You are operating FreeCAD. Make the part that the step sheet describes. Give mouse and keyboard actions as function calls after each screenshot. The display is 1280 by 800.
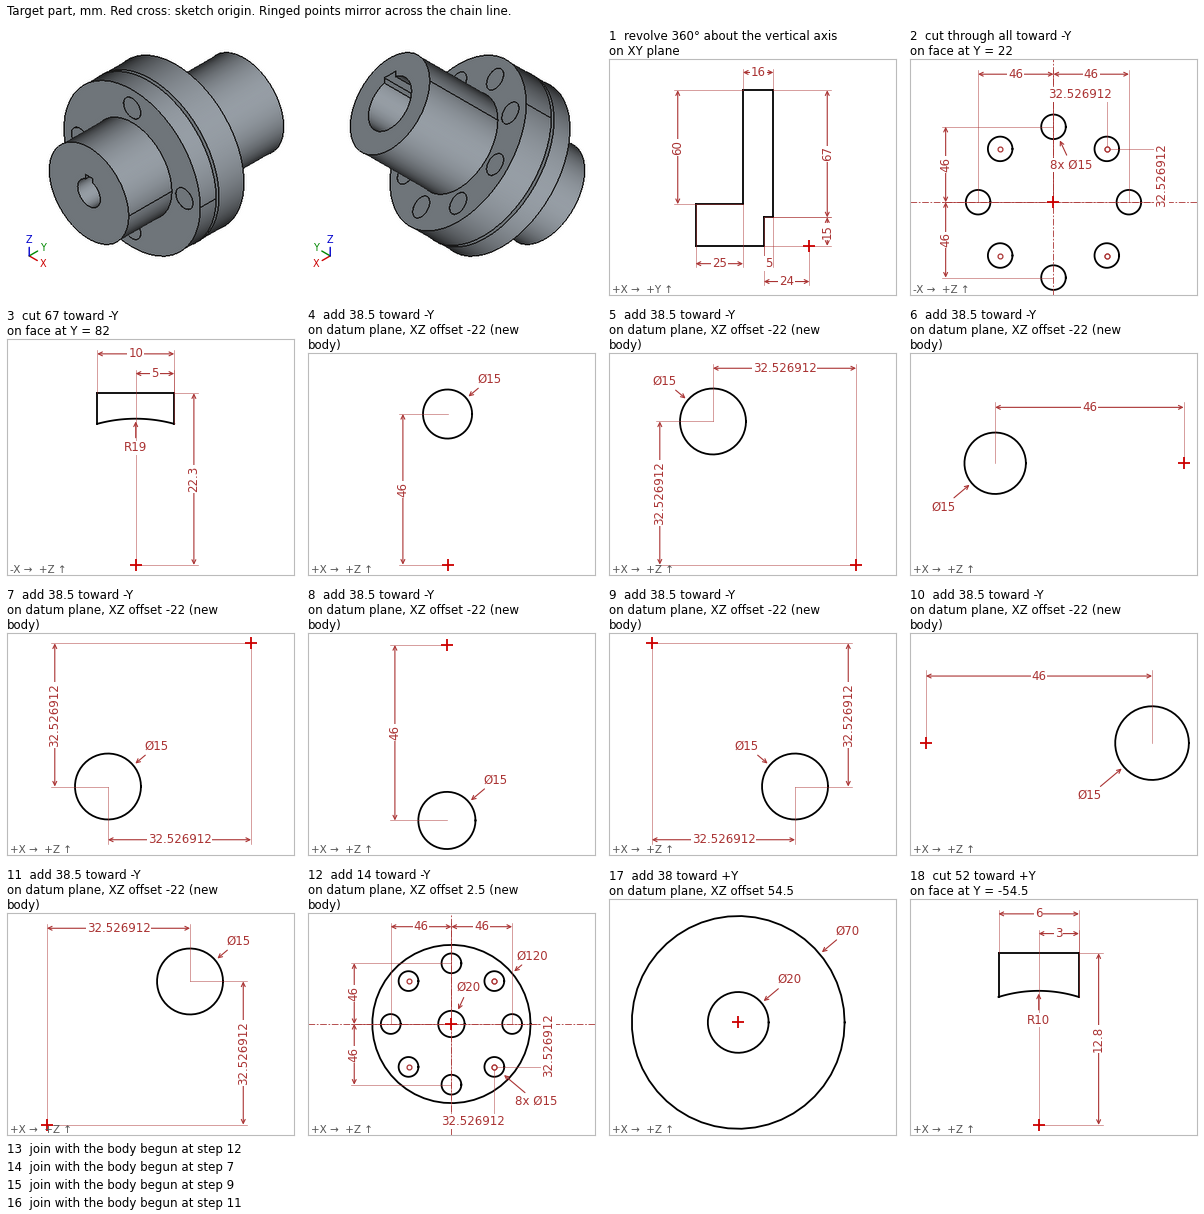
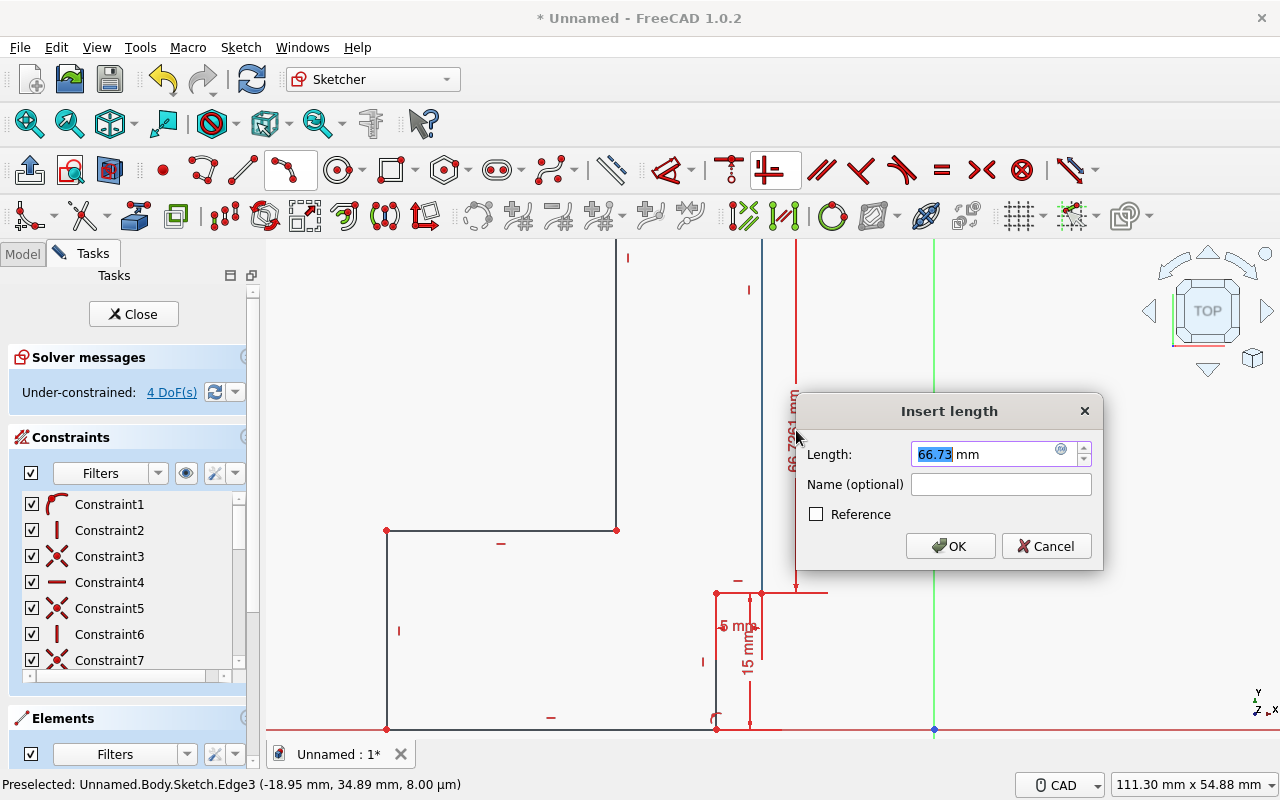
text(67)
key(Return)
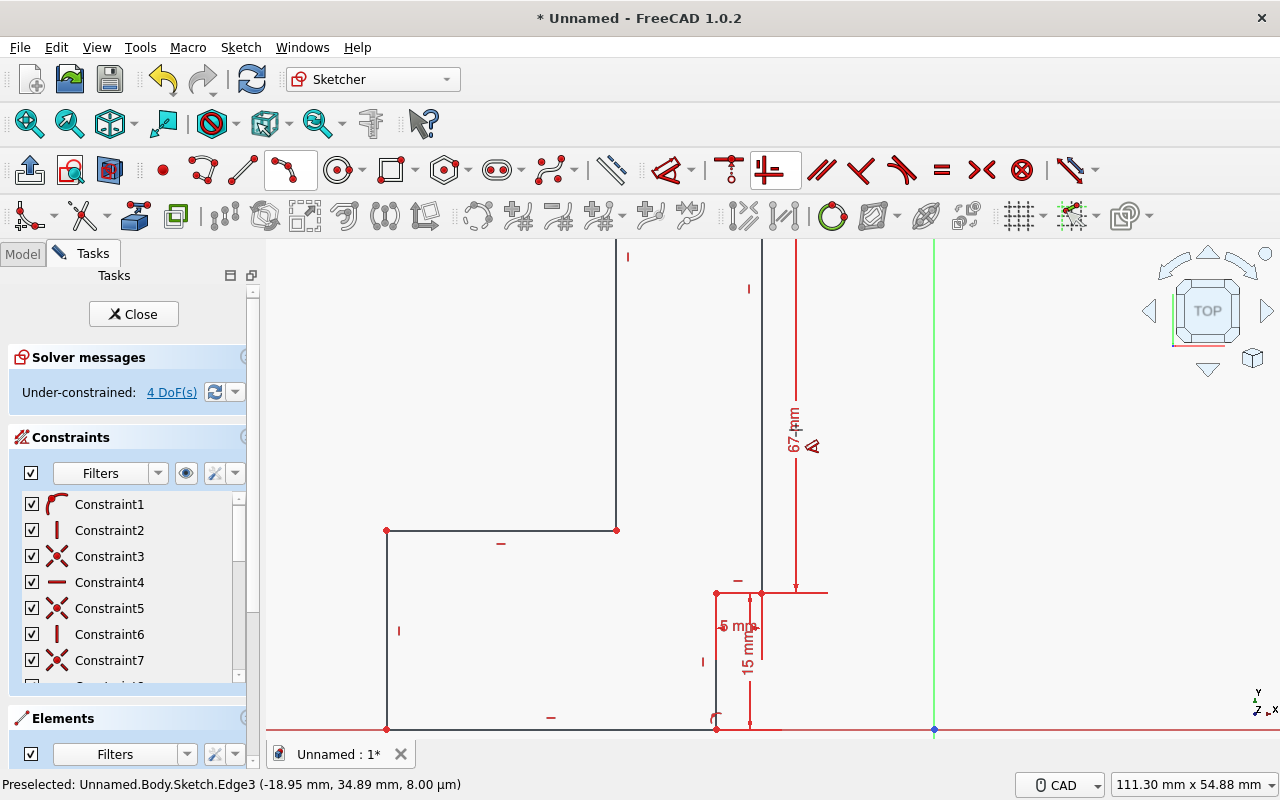
scroll(740, 597, down, 4)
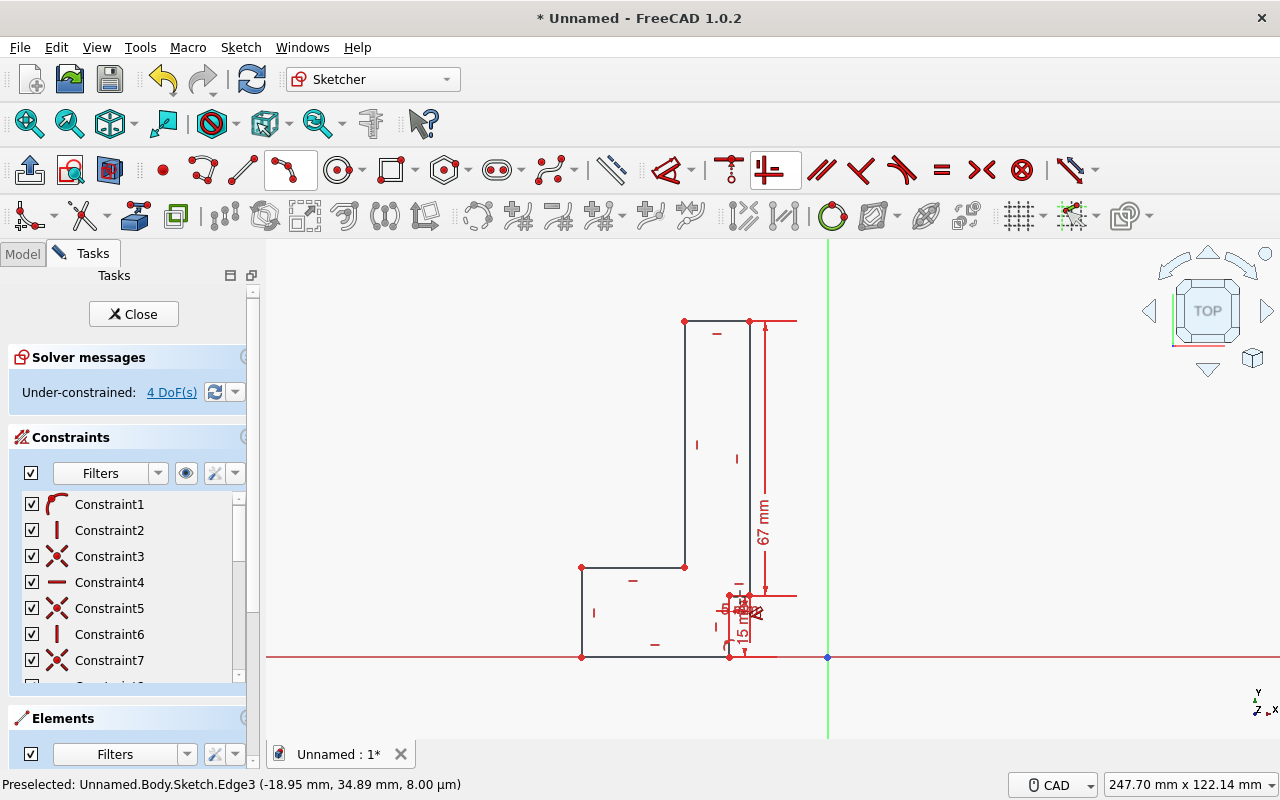
click(730, 321)
click(717, 287)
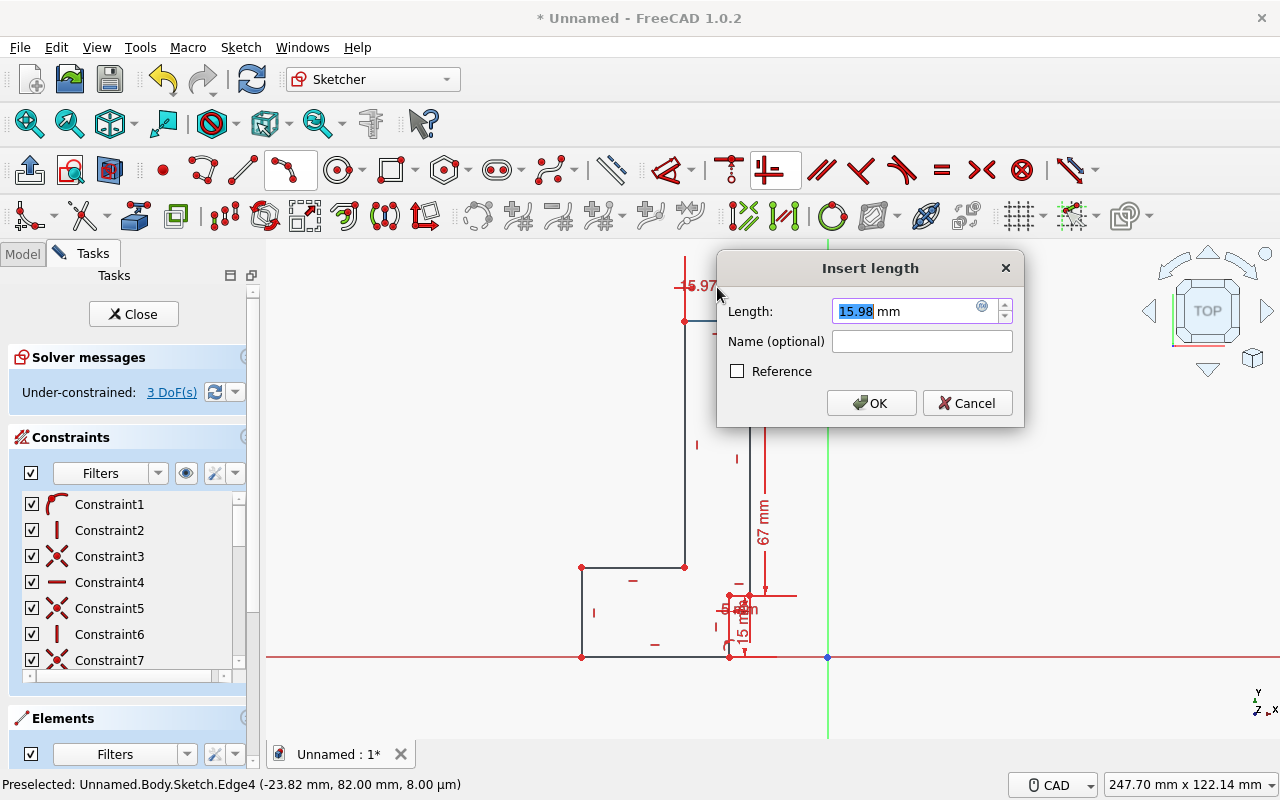
text(16)
key(Return)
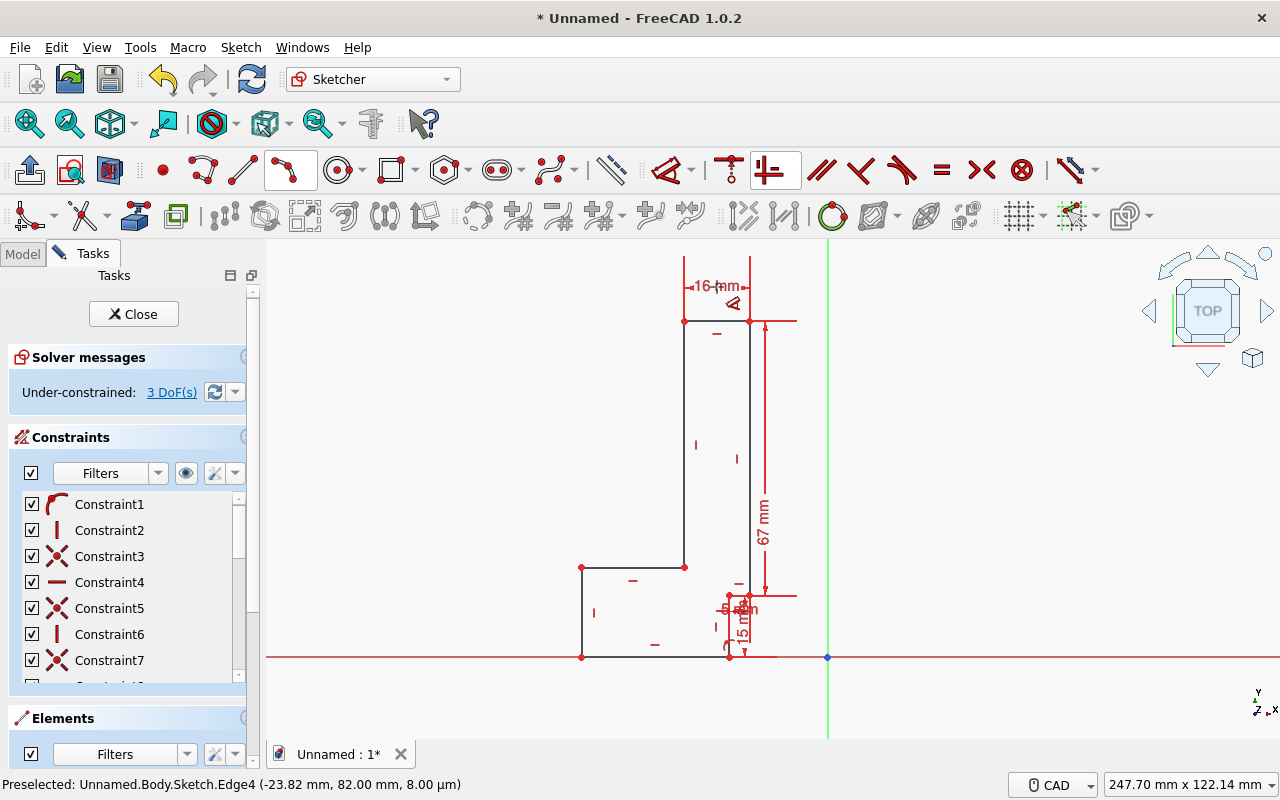
click(684, 395)
click(650, 444)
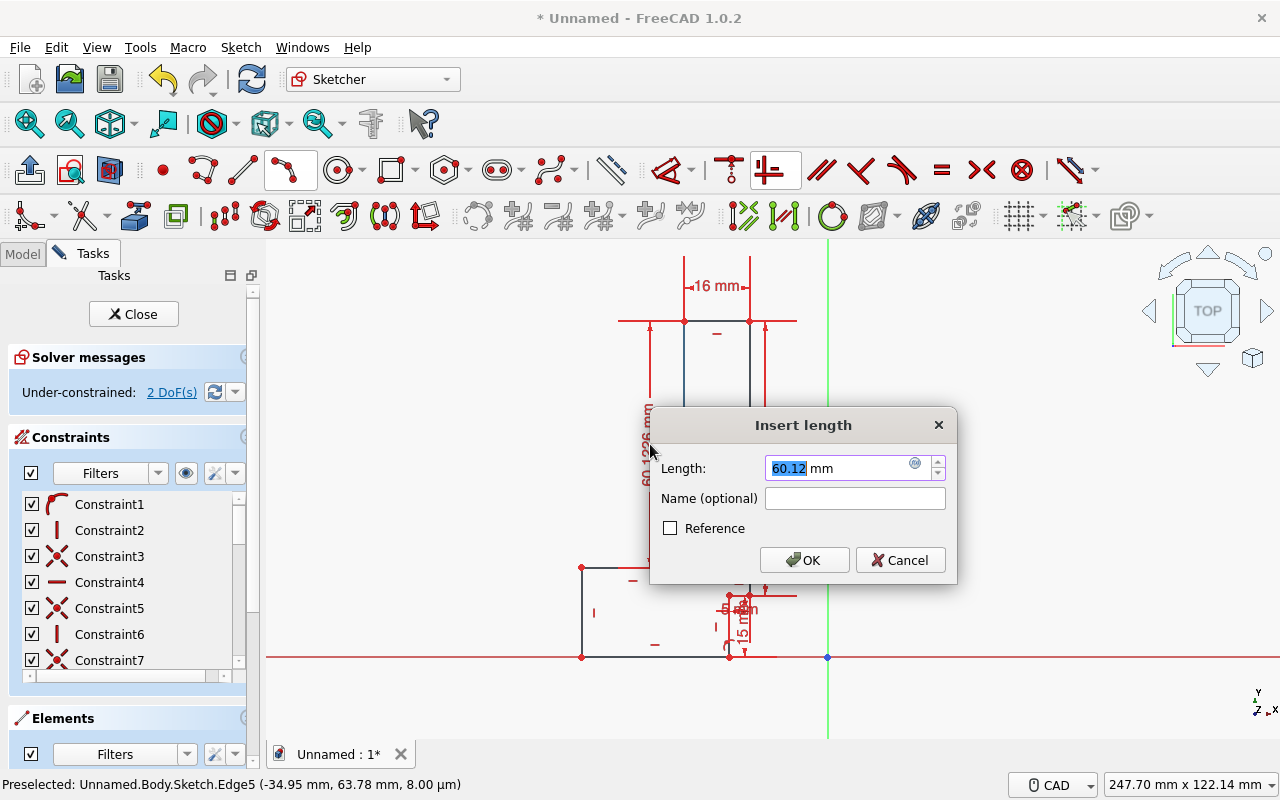
text(60)
key(Return)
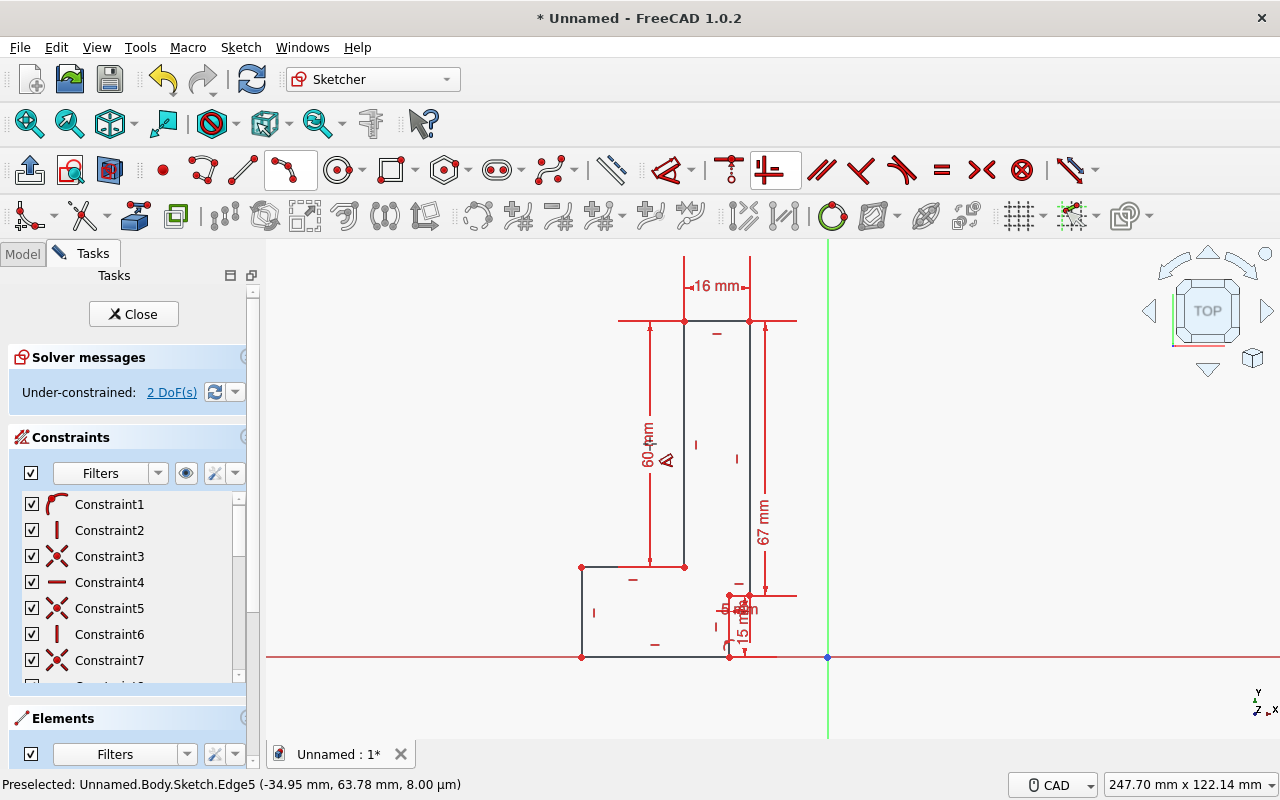
click(654, 567)
click(633, 601)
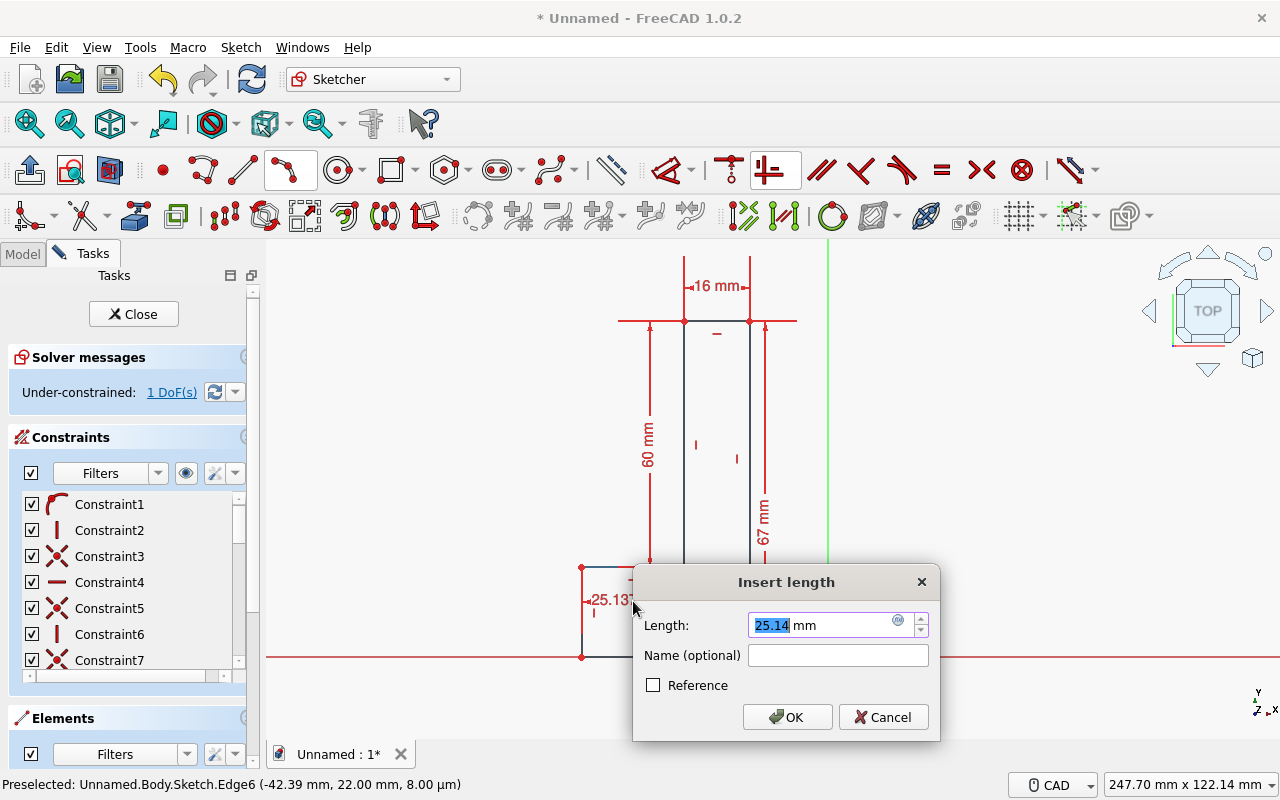
text(25)
key(Return)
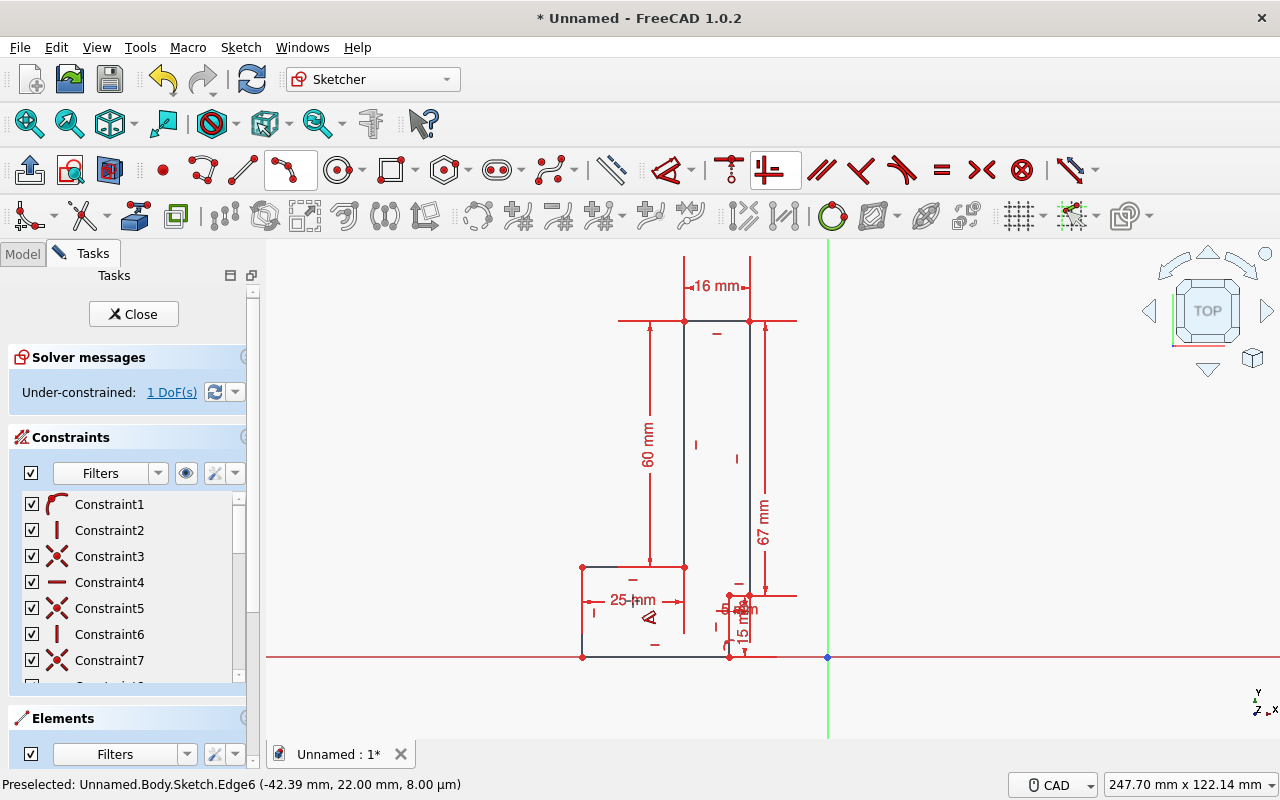
click(729, 657)
click(779, 691)